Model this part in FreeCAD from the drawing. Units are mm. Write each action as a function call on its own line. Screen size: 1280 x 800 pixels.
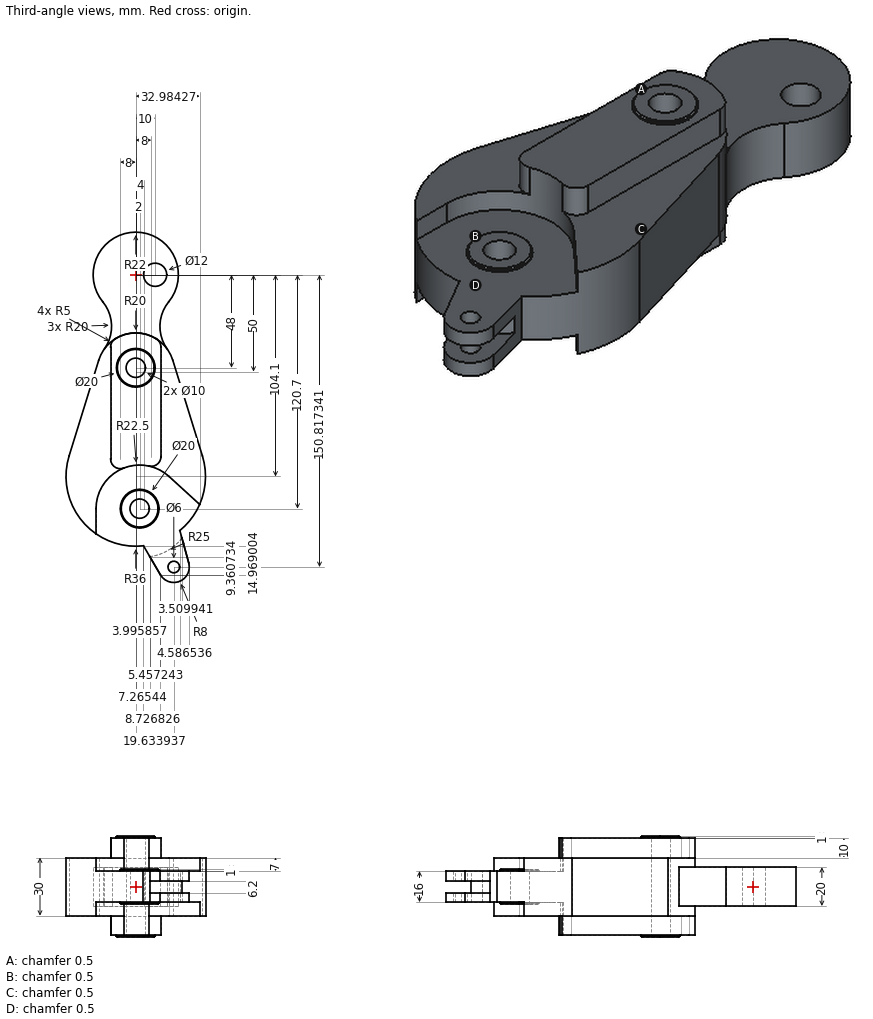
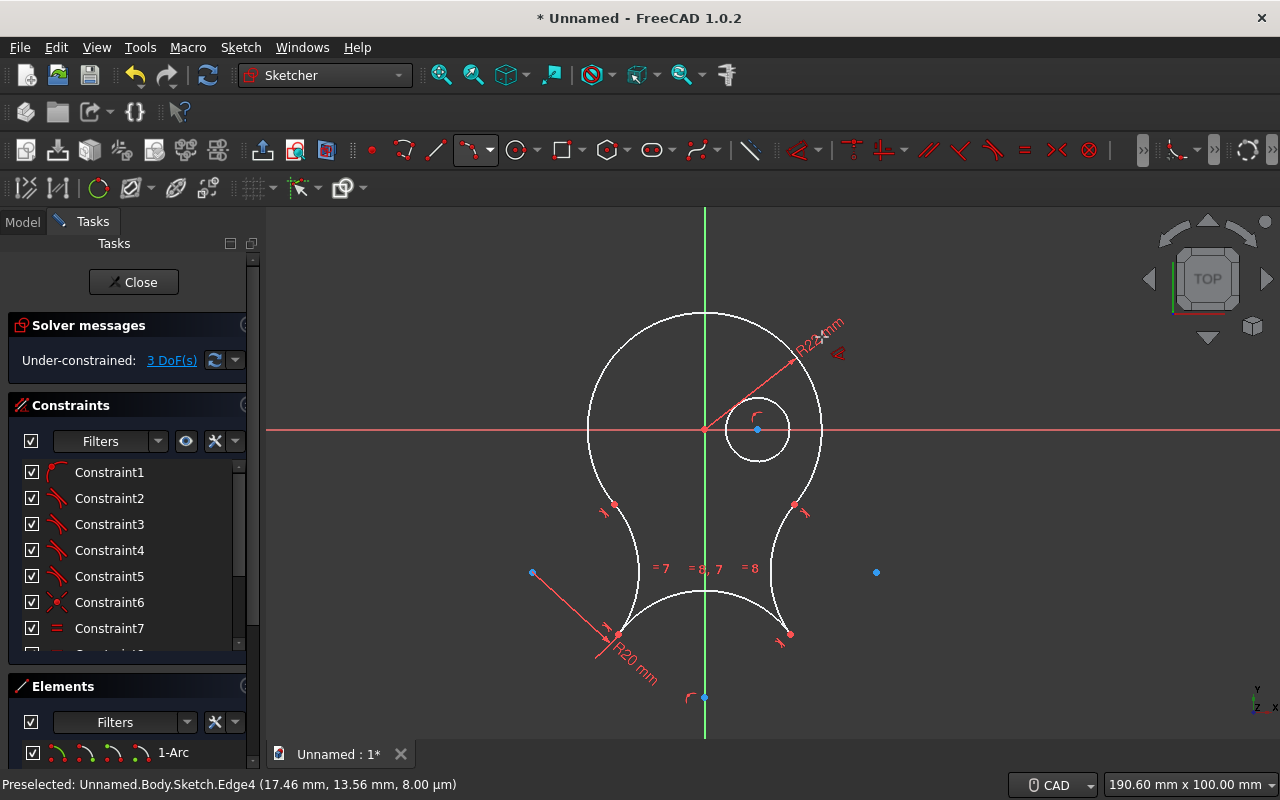
click(780, 407)
click(775, 368)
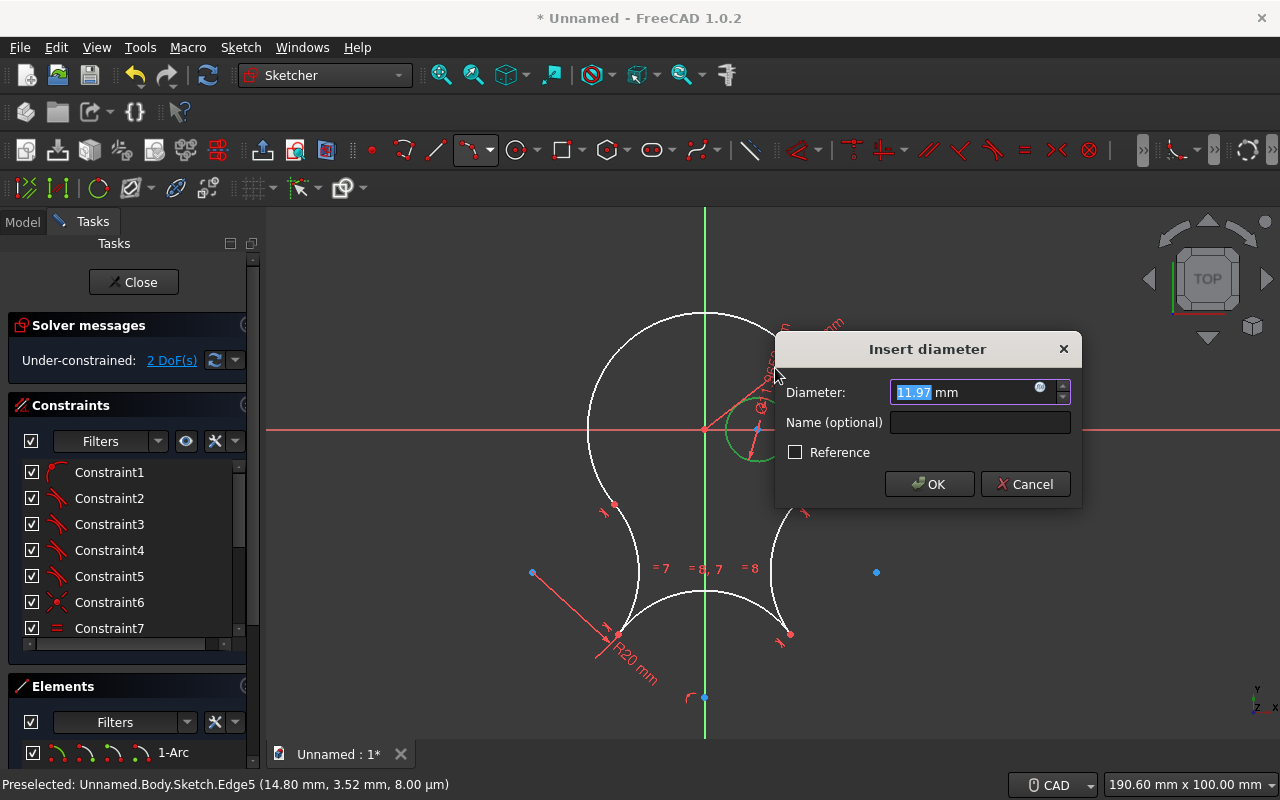
text(12)
key(Return)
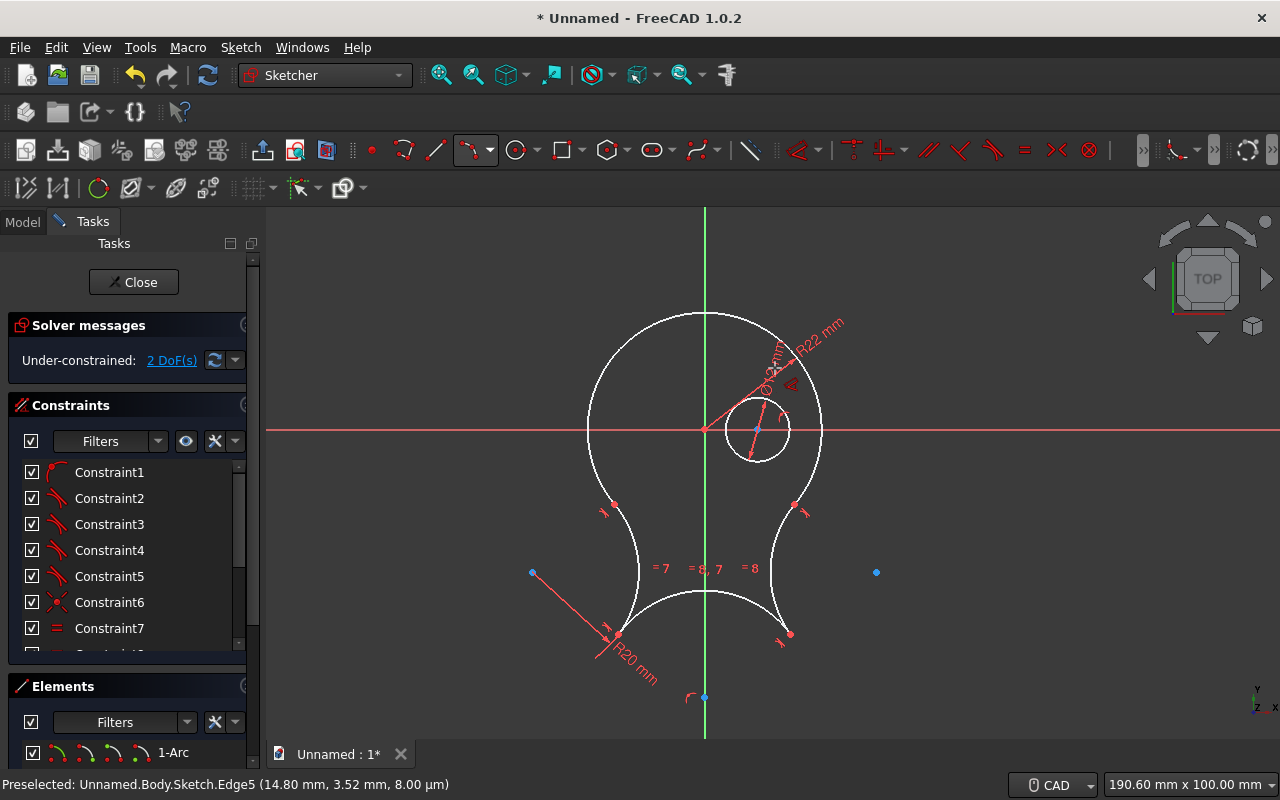
click(758, 430)
click(719, 396)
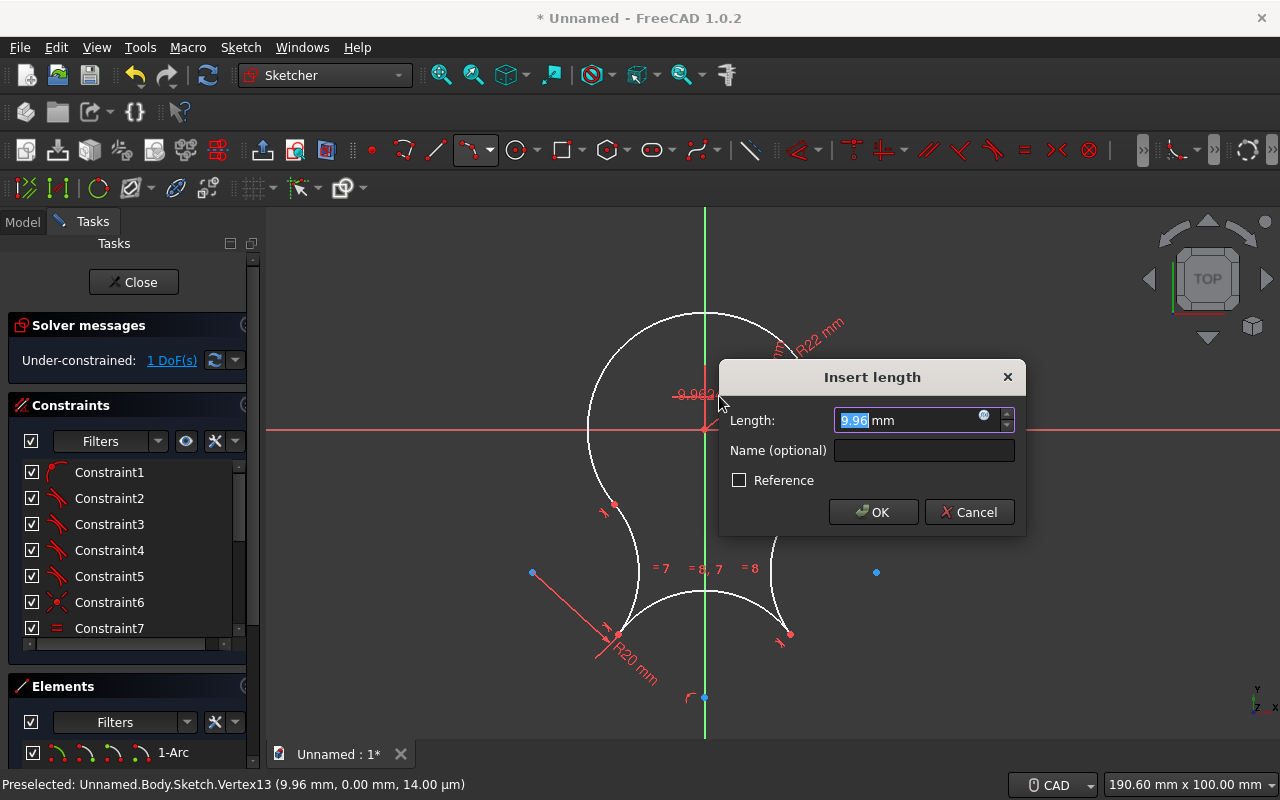
text(10)
key(Return)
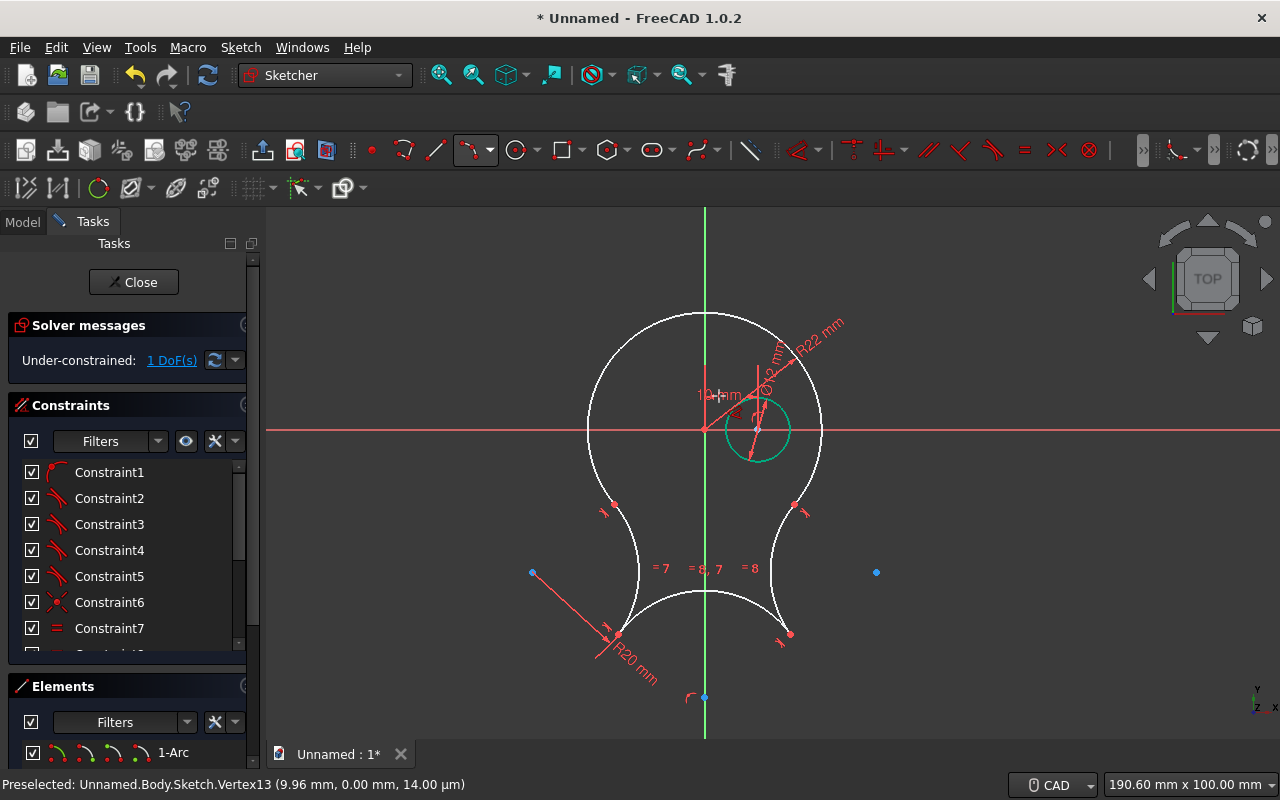
click(705, 697)
click(739, 563)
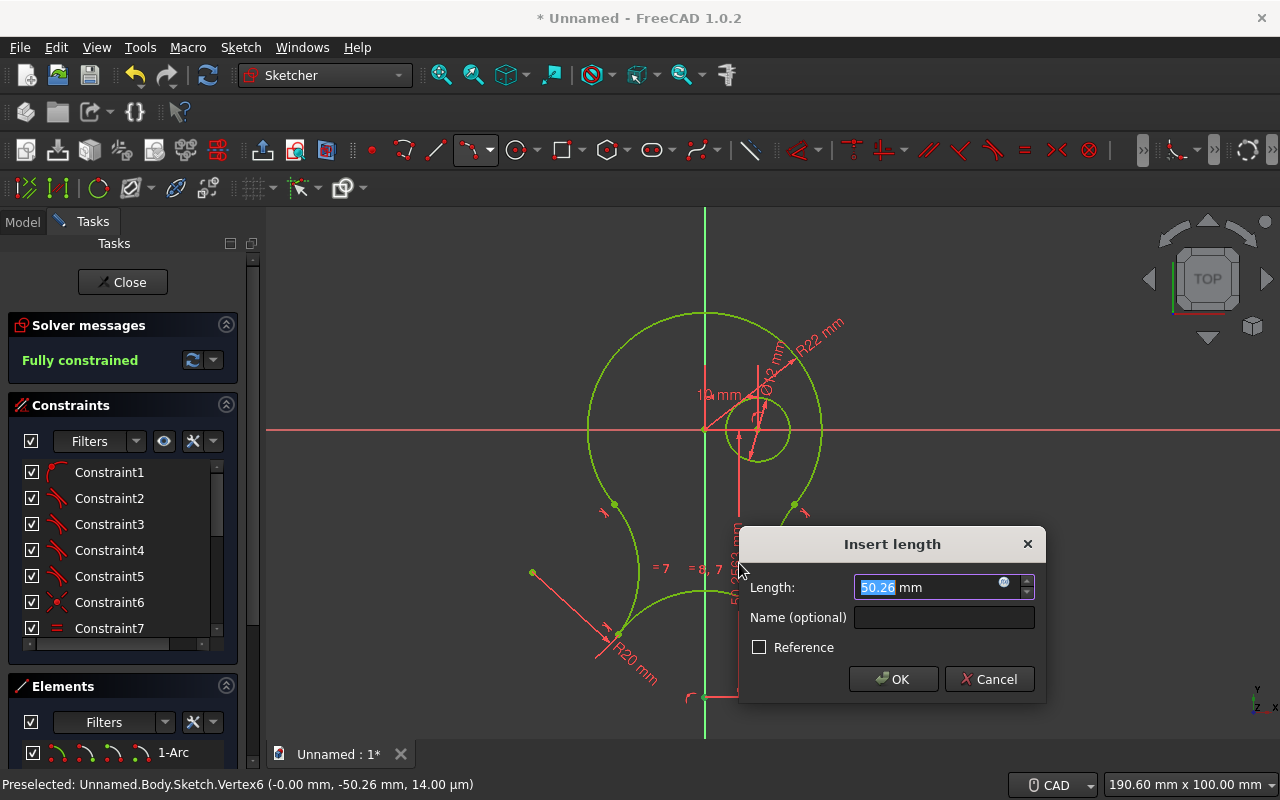
text(50)
key(Return)
key(Escape)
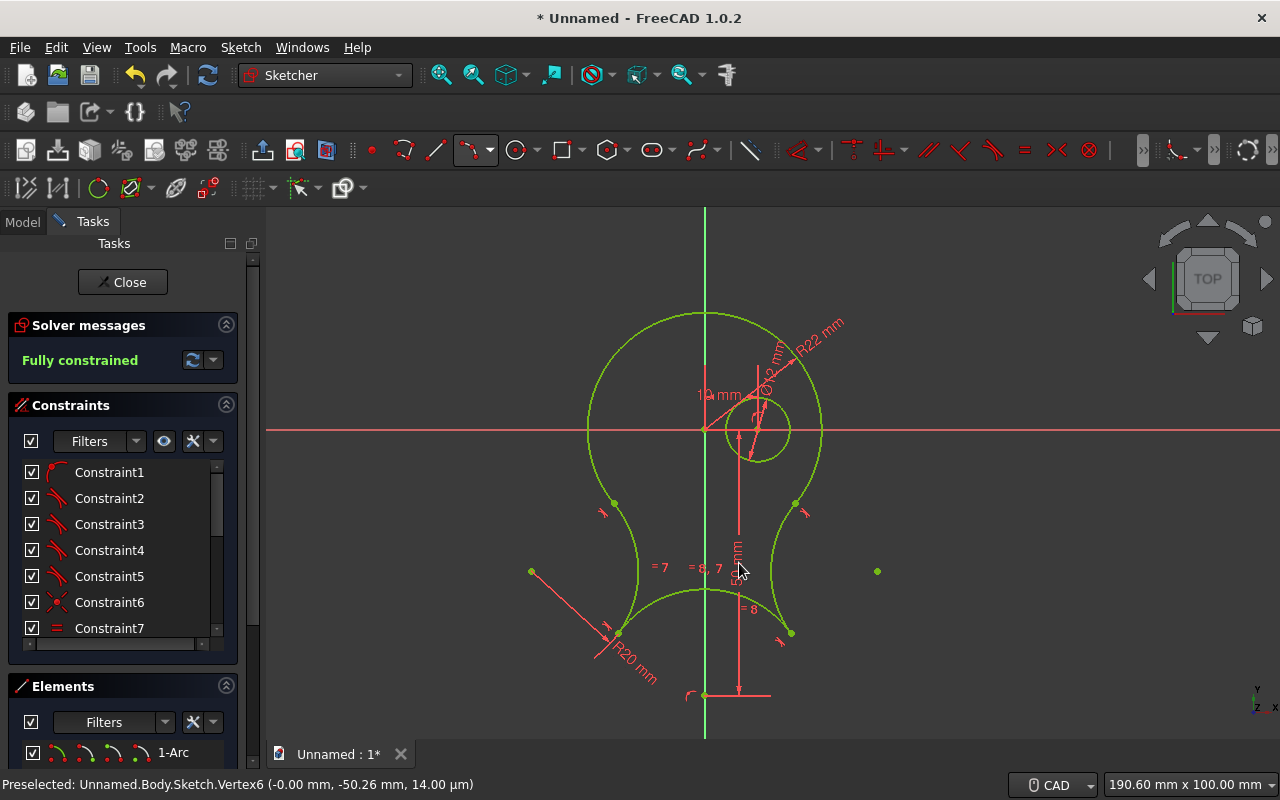
click(123, 282)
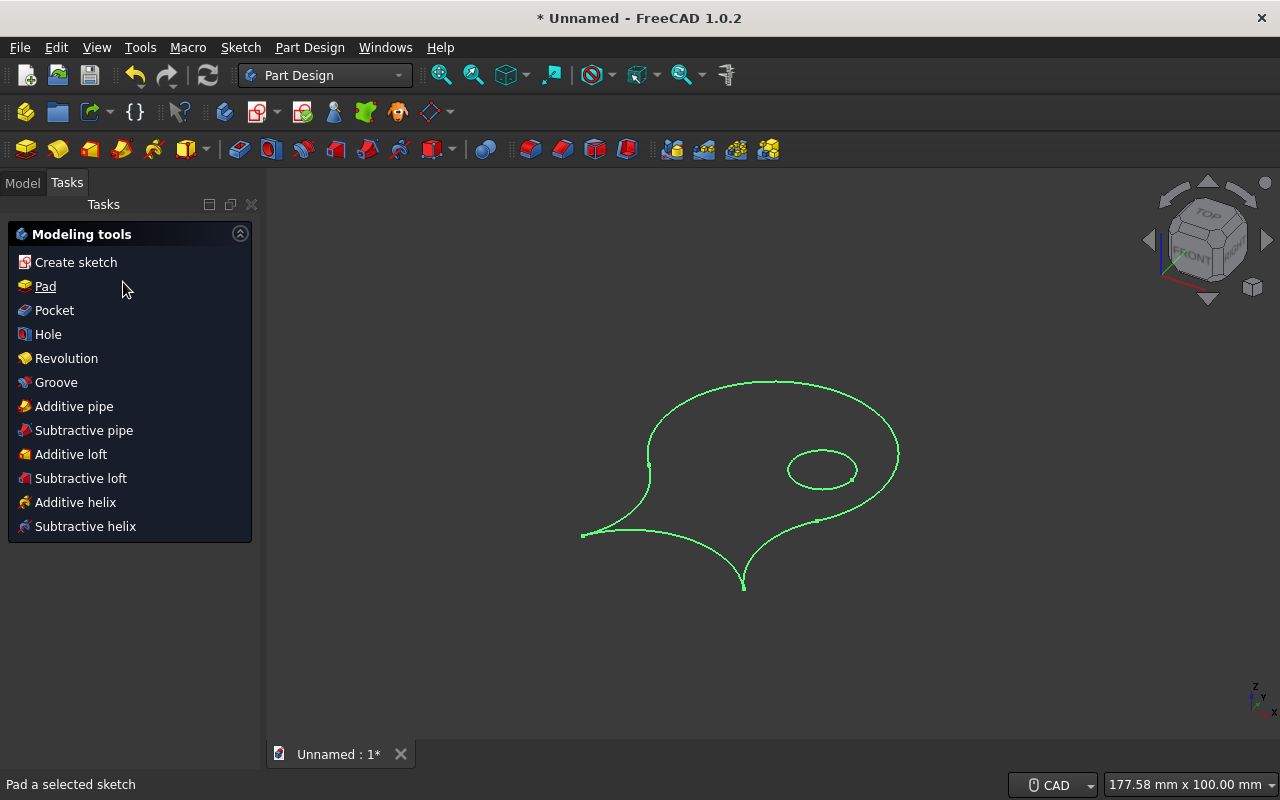
click(26, 150)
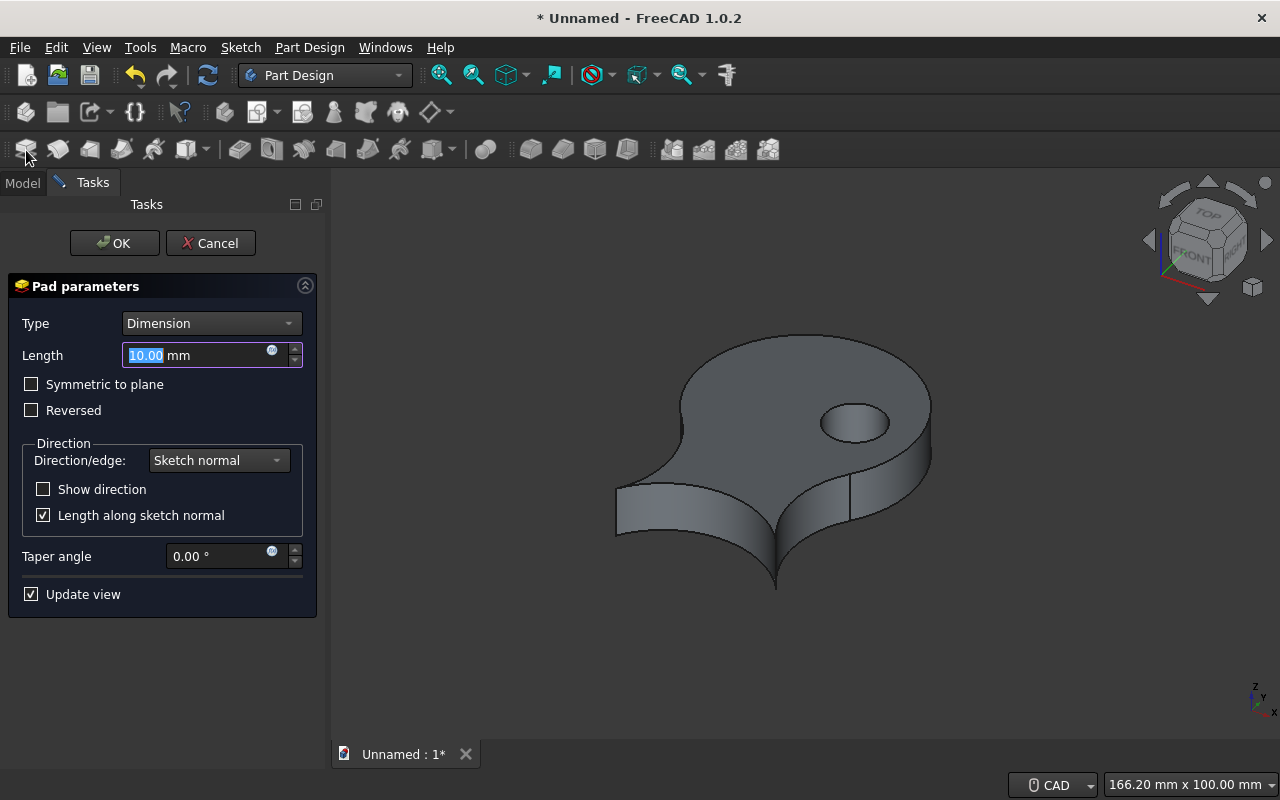
text(20)
key(Tab)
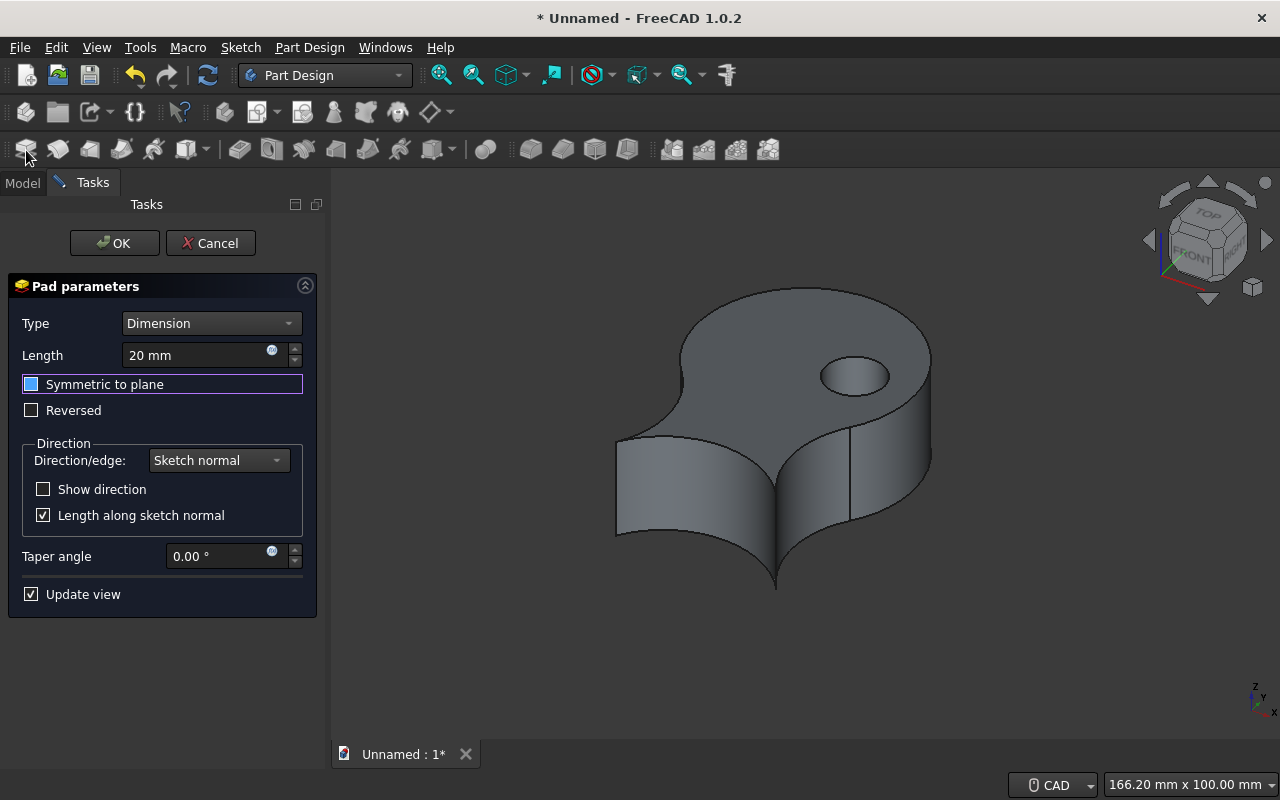
click(30, 384)